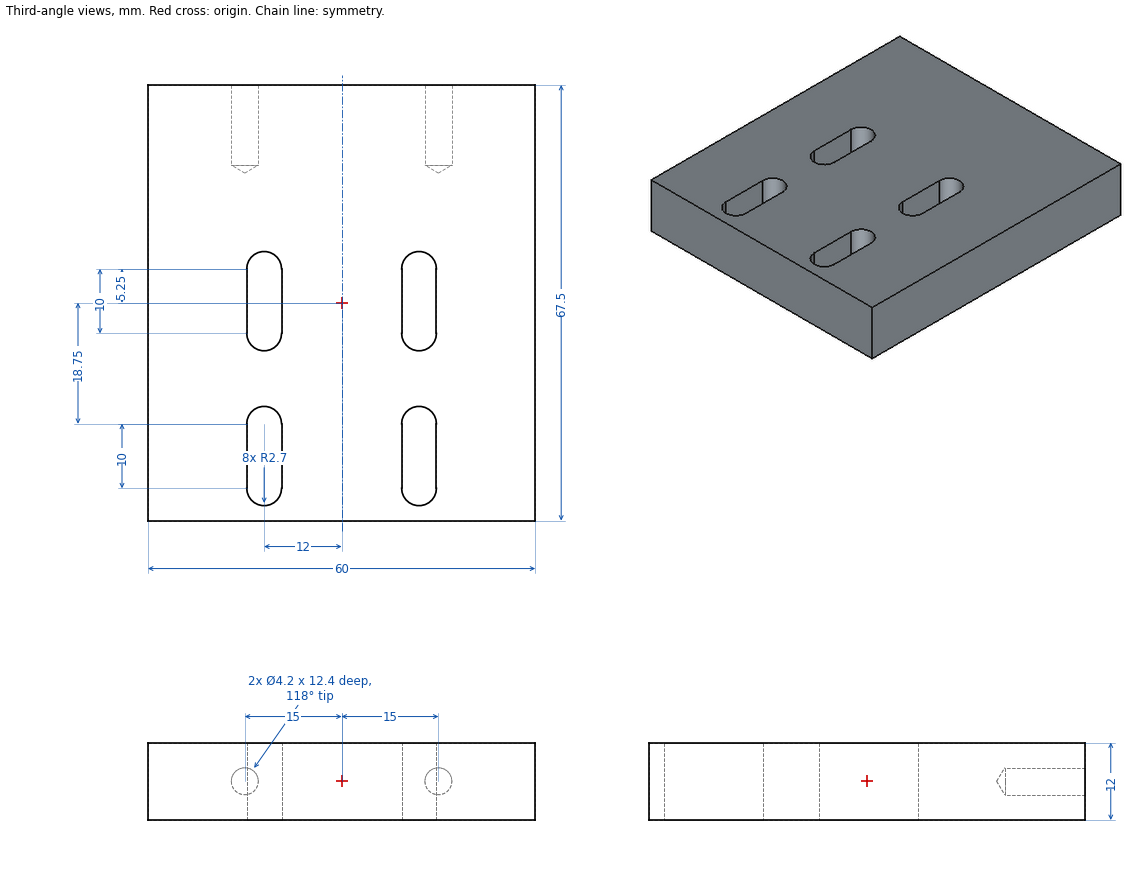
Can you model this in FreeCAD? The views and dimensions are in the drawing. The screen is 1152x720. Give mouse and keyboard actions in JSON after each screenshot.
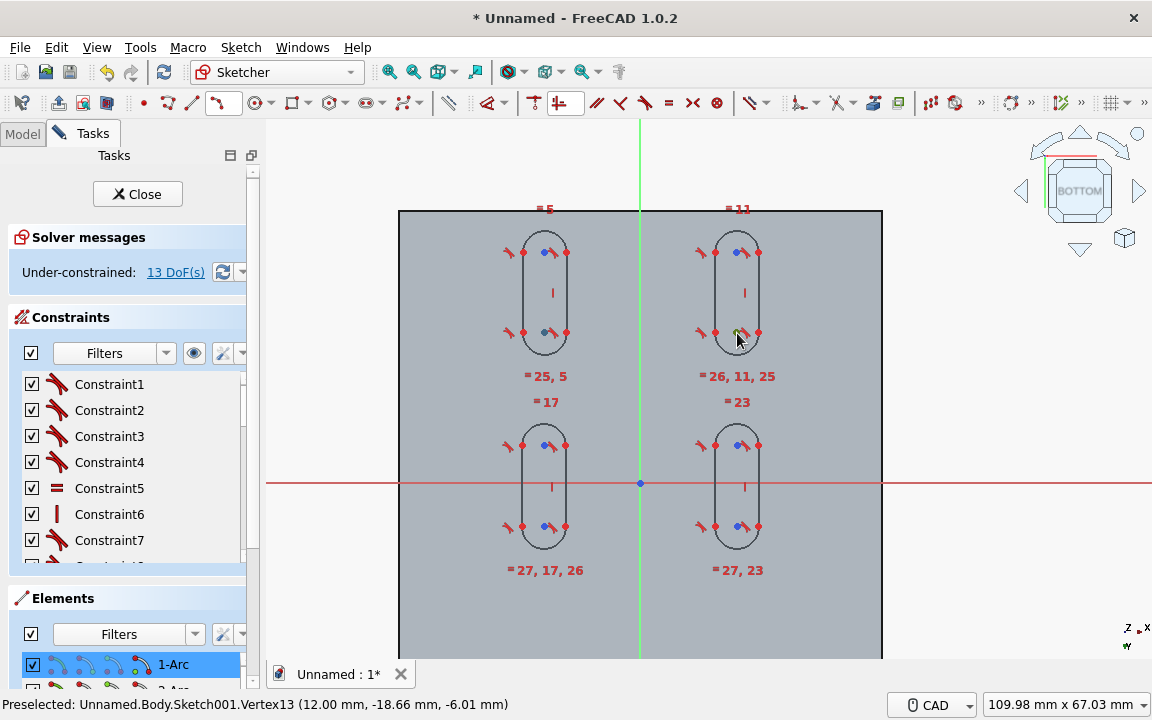
{"action": "left_click", "coordinate": [640, 596]}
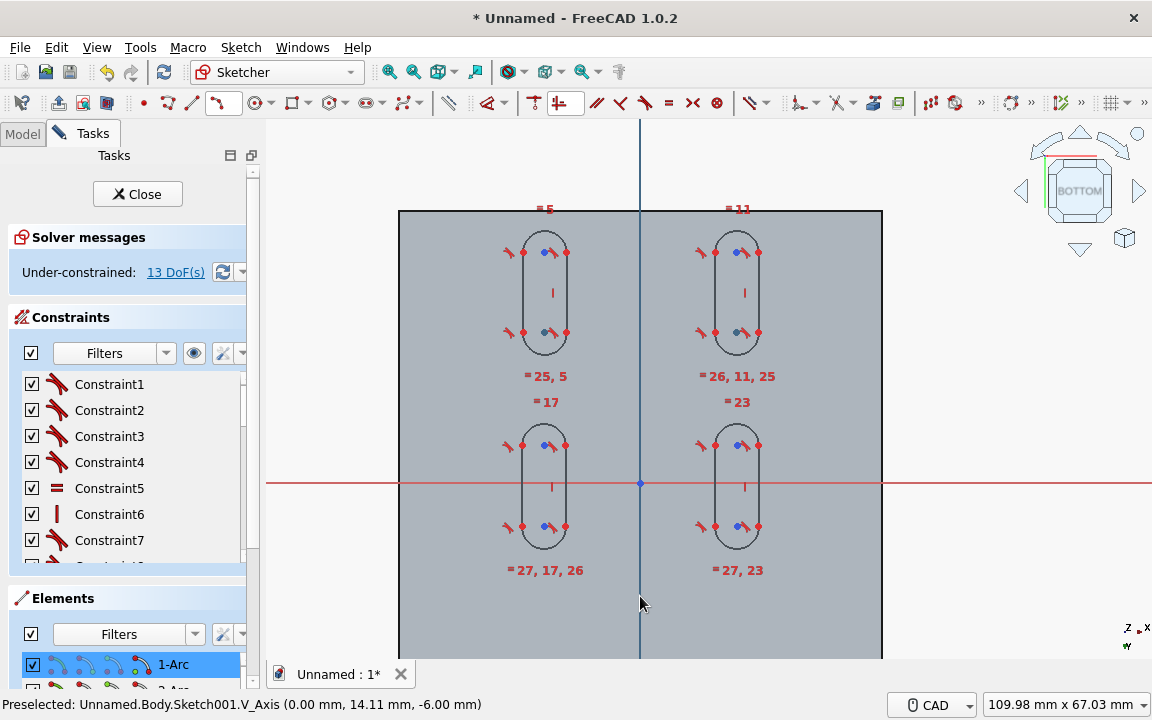
{"action": "key", "text": "s"}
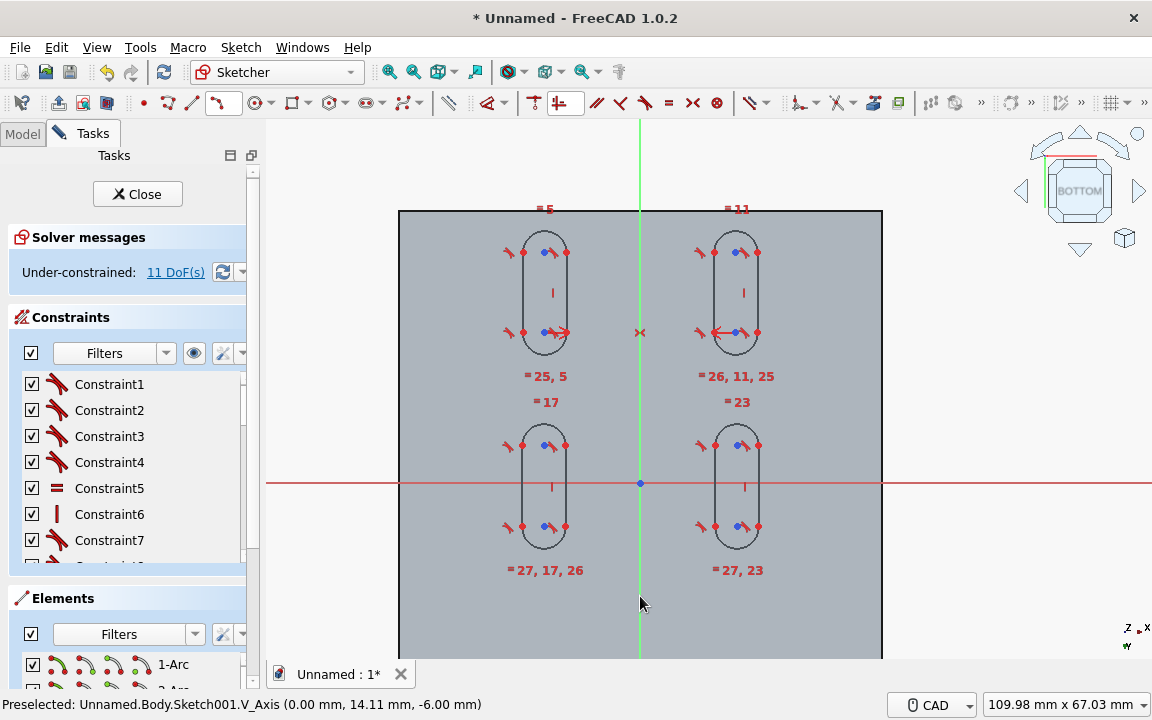
{"action": "left_click", "coordinate": [544, 527]}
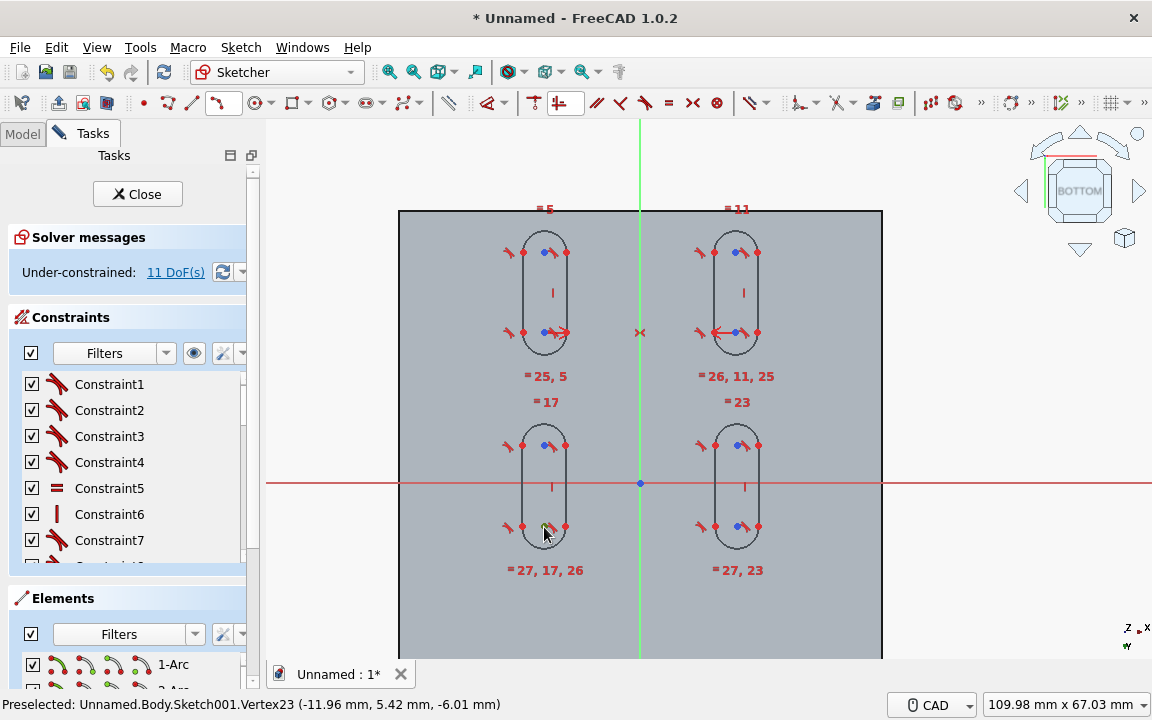
{"action": "left_click", "coordinate": [737, 527]}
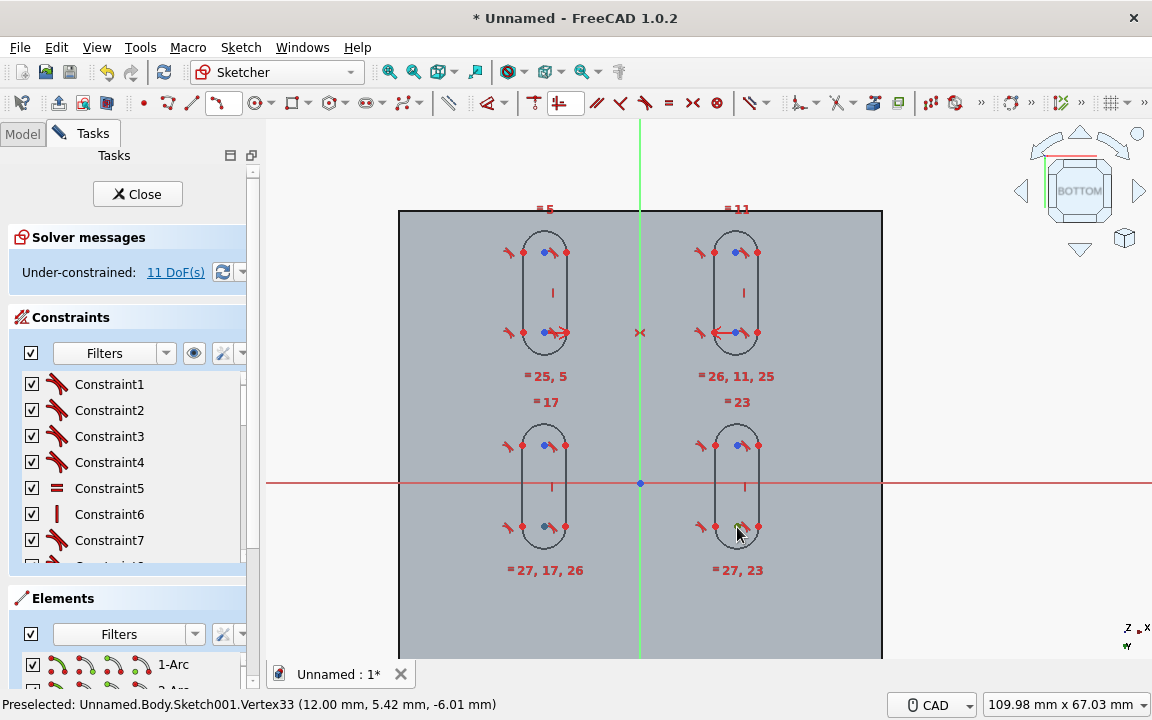
{"action": "left_click", "coordinate": [640, 596]}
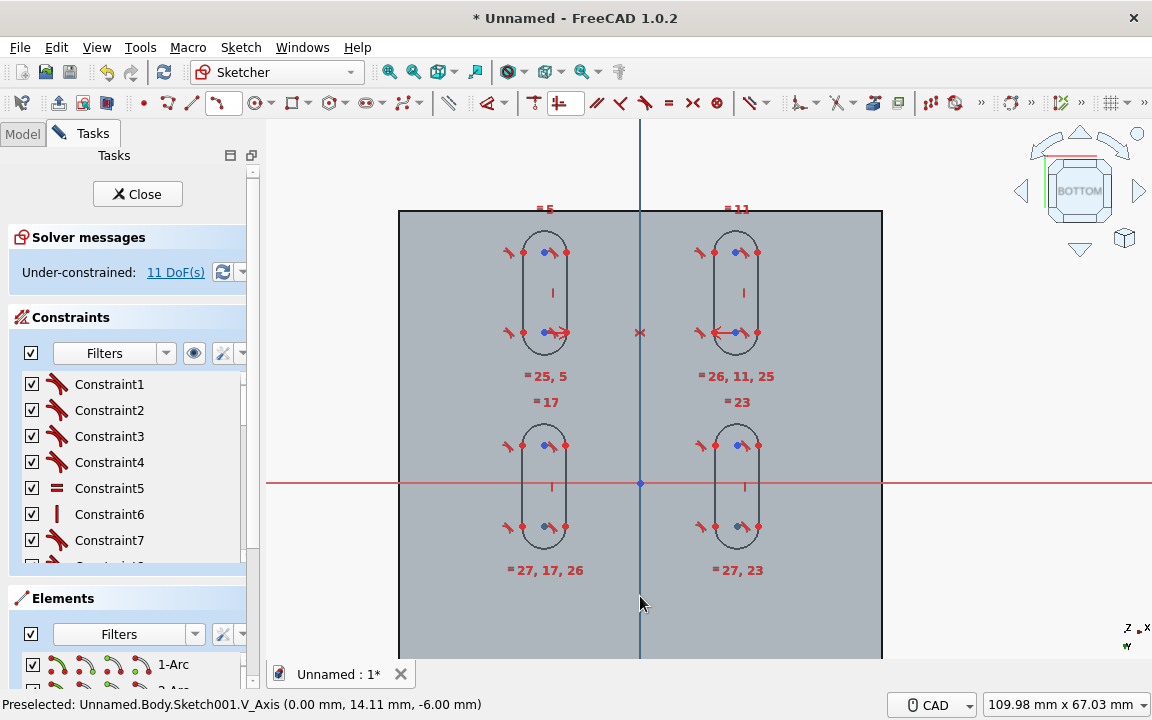
{"action": "key", "text": "s"}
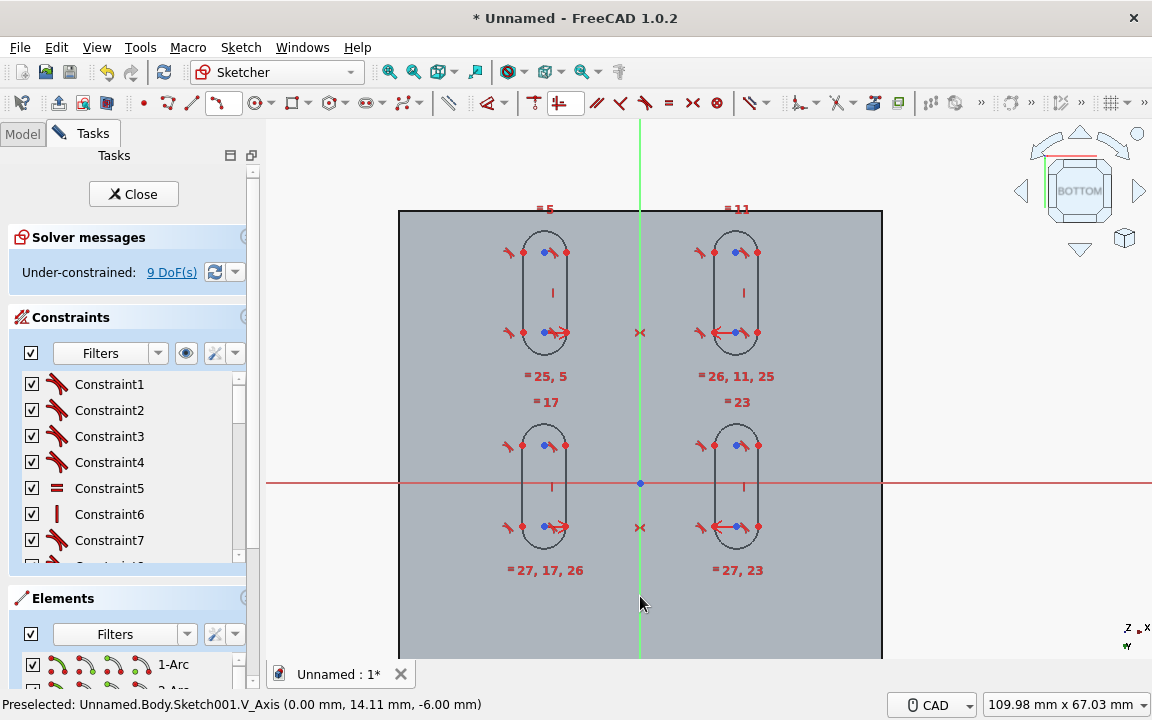
{"action": "scroll", "coordinate": [532, 351], "scroll_direction": "up", "scroll_amount": 4}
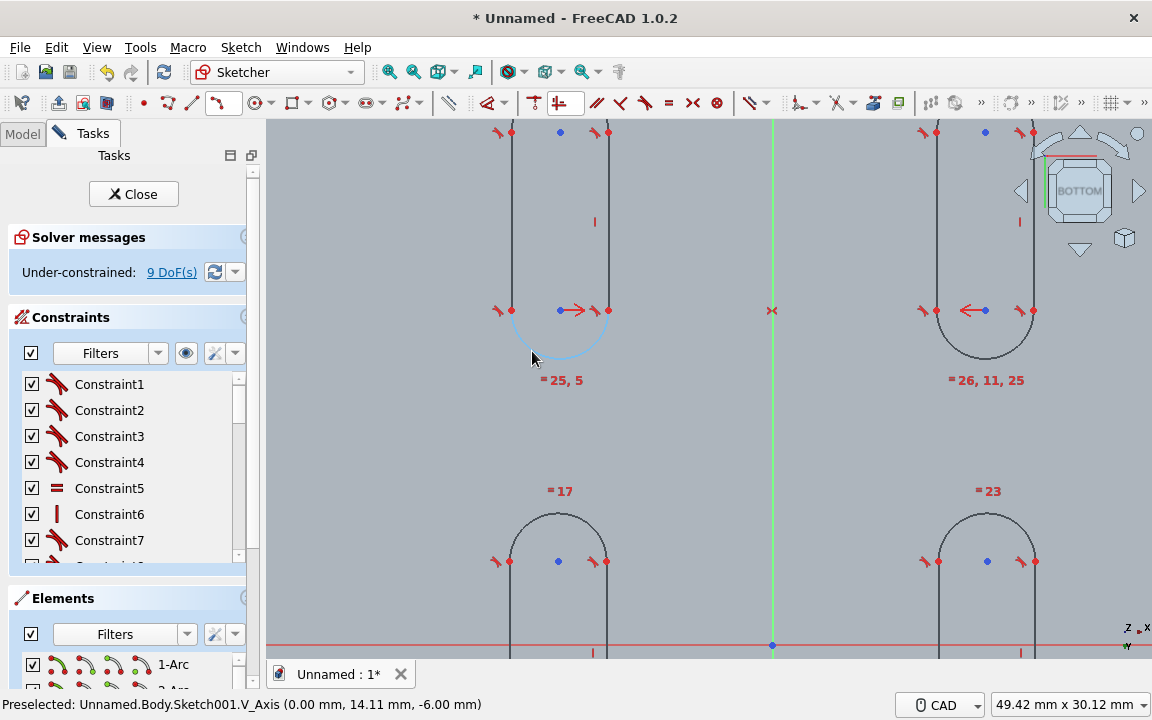
{"action": "left_click", "coordinate": [532, 350]}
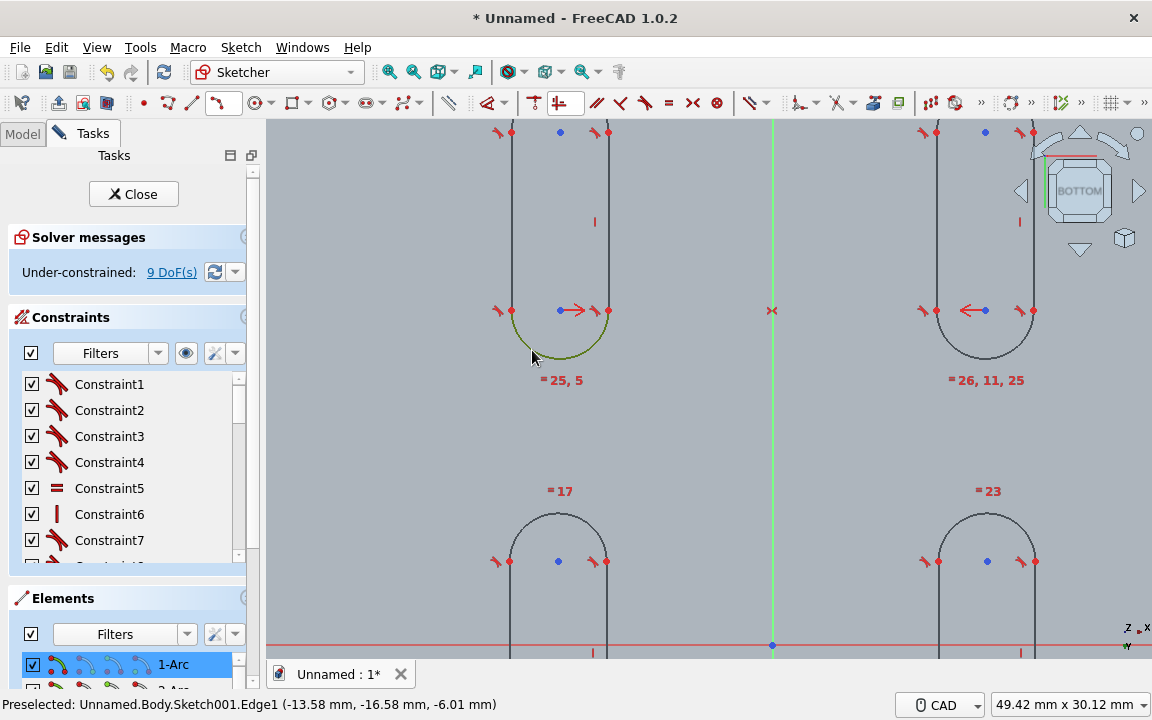
{"action": "key", "text": "k r"}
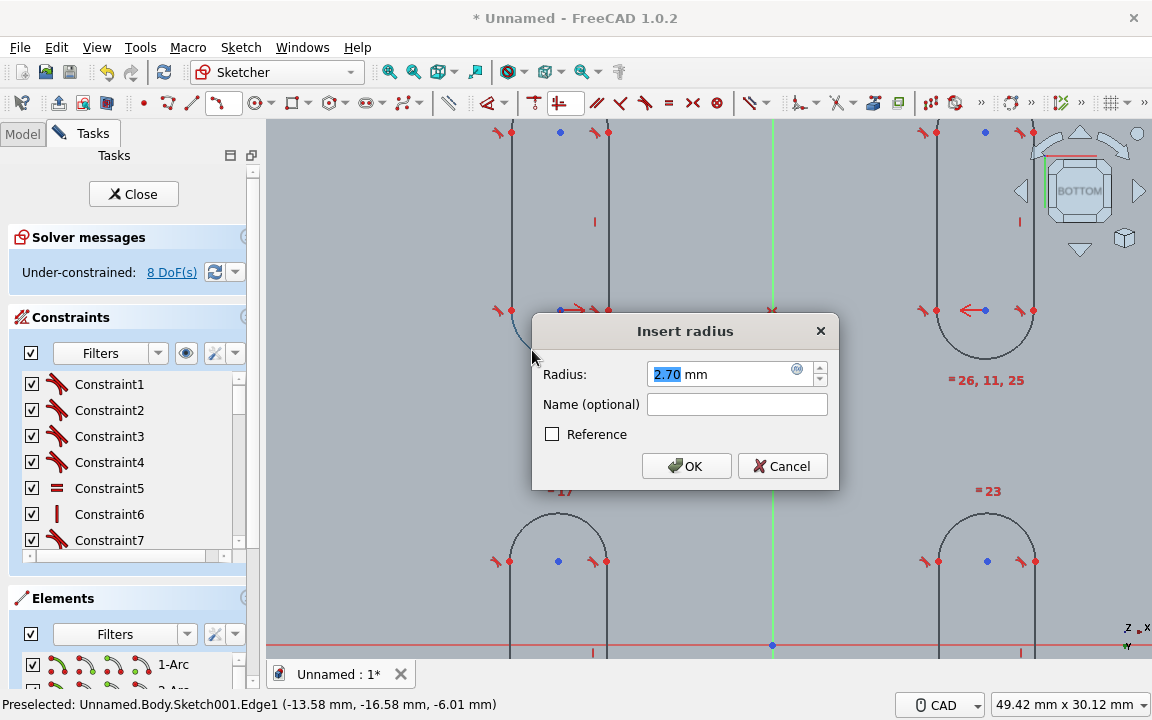
{"action": "type", "text": "2.7"}
{"action": "key", "text": "Return"}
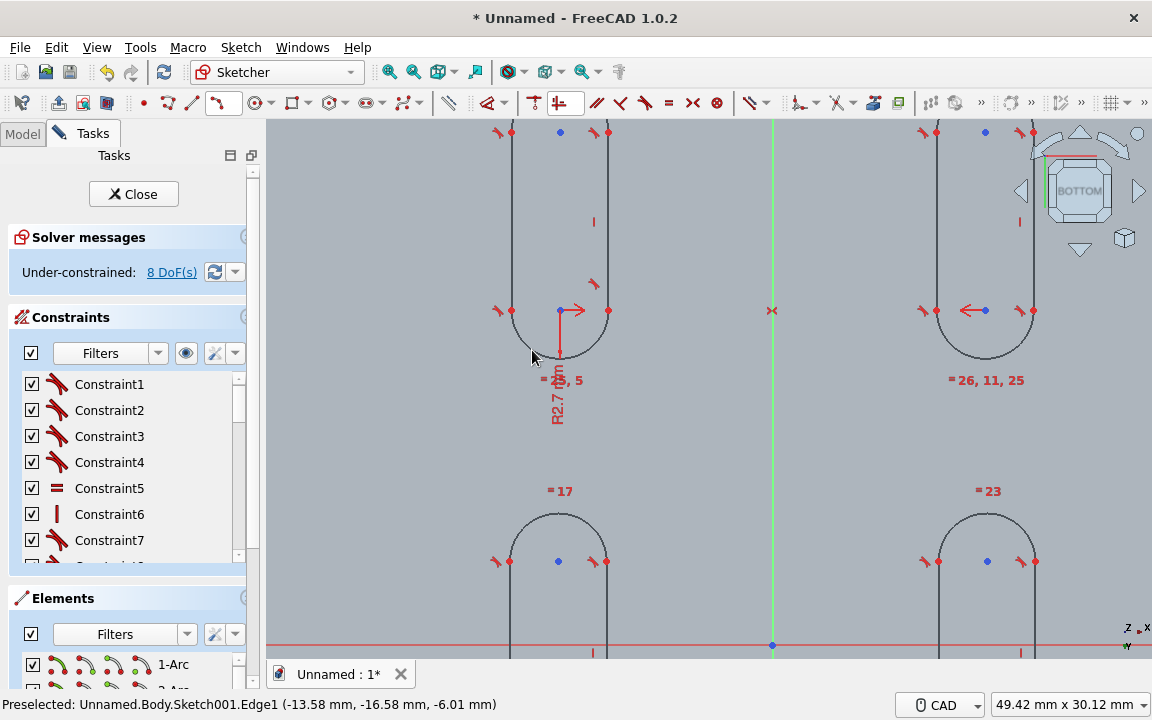
{"action": "left_click", "coordinate": [512, 257]}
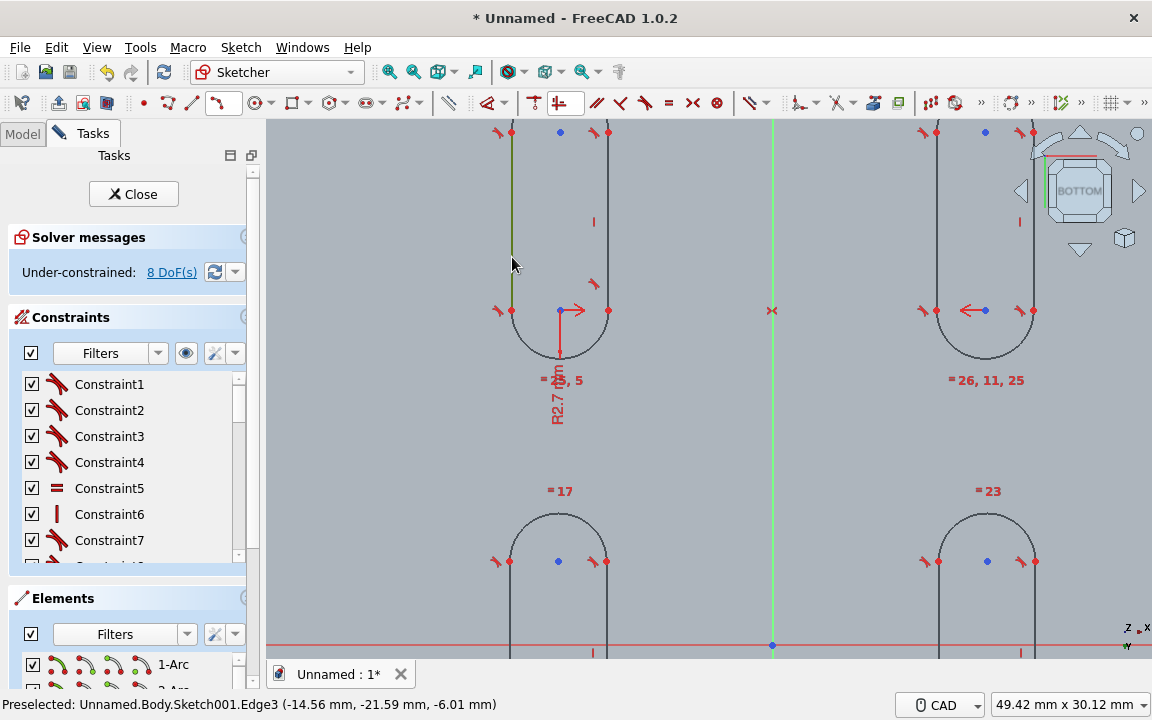
{"action": "key", "text": "i"}